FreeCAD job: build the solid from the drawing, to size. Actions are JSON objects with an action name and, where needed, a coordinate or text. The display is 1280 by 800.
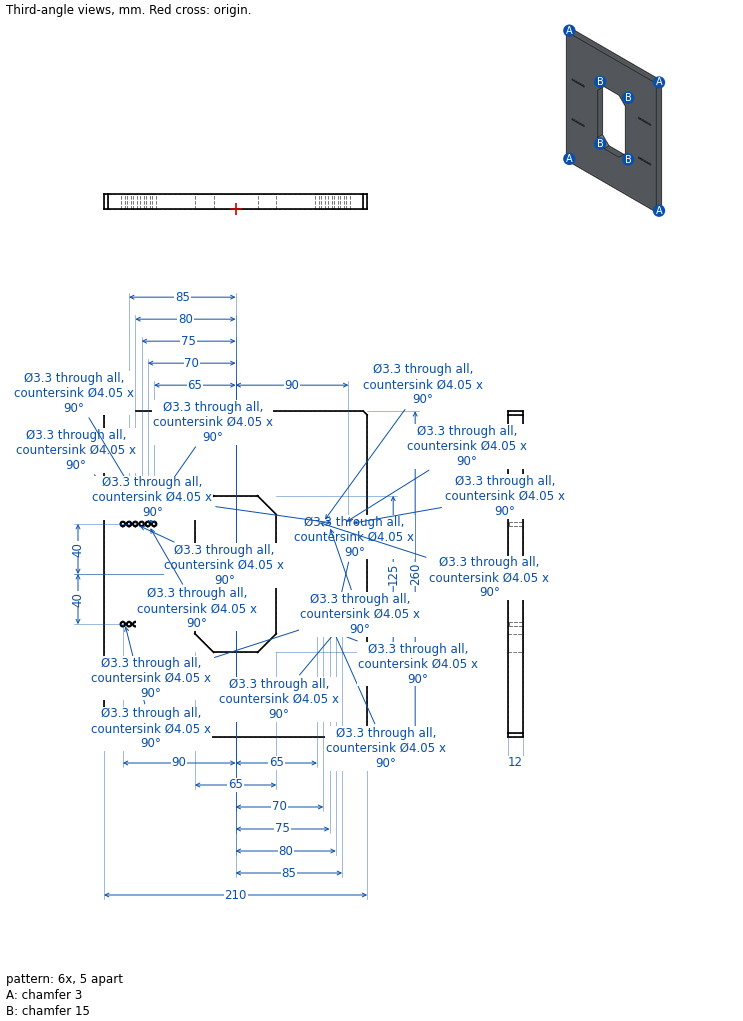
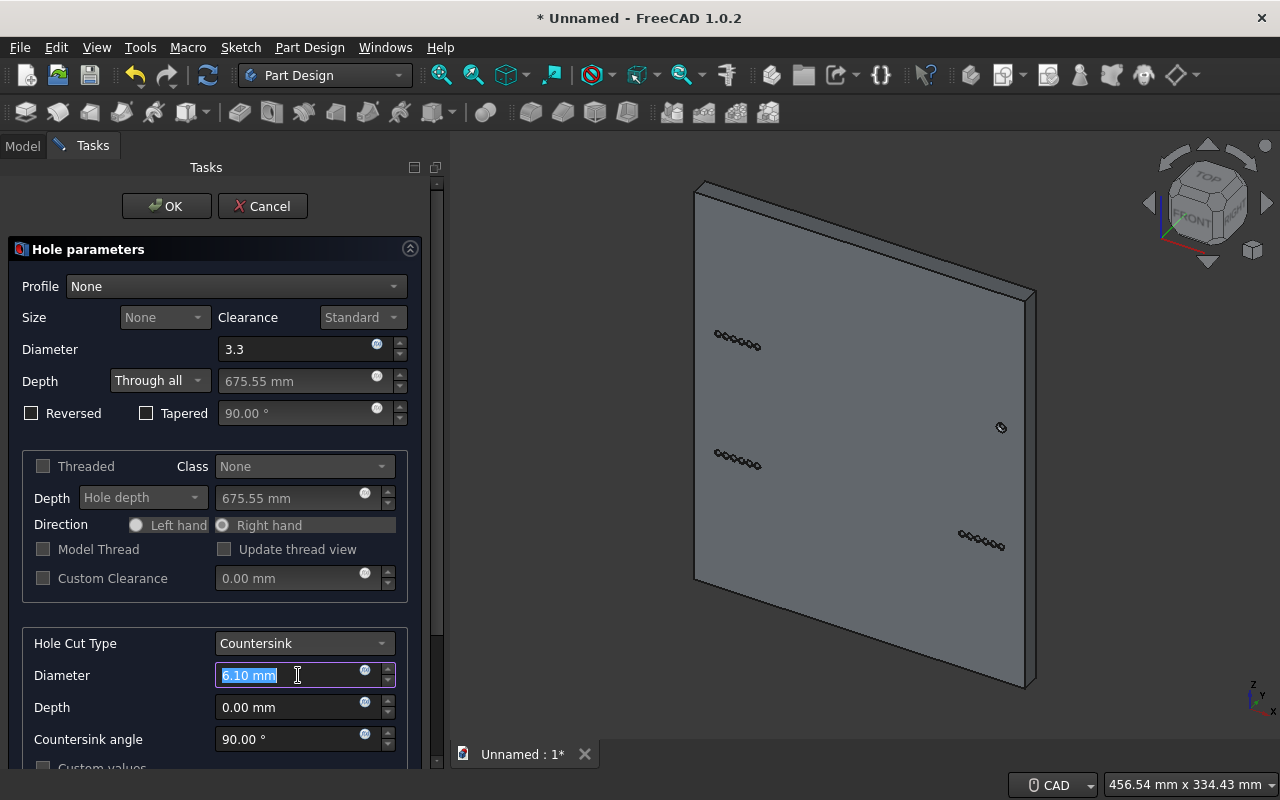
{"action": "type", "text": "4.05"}
{"action": "key", "text": "Tab"}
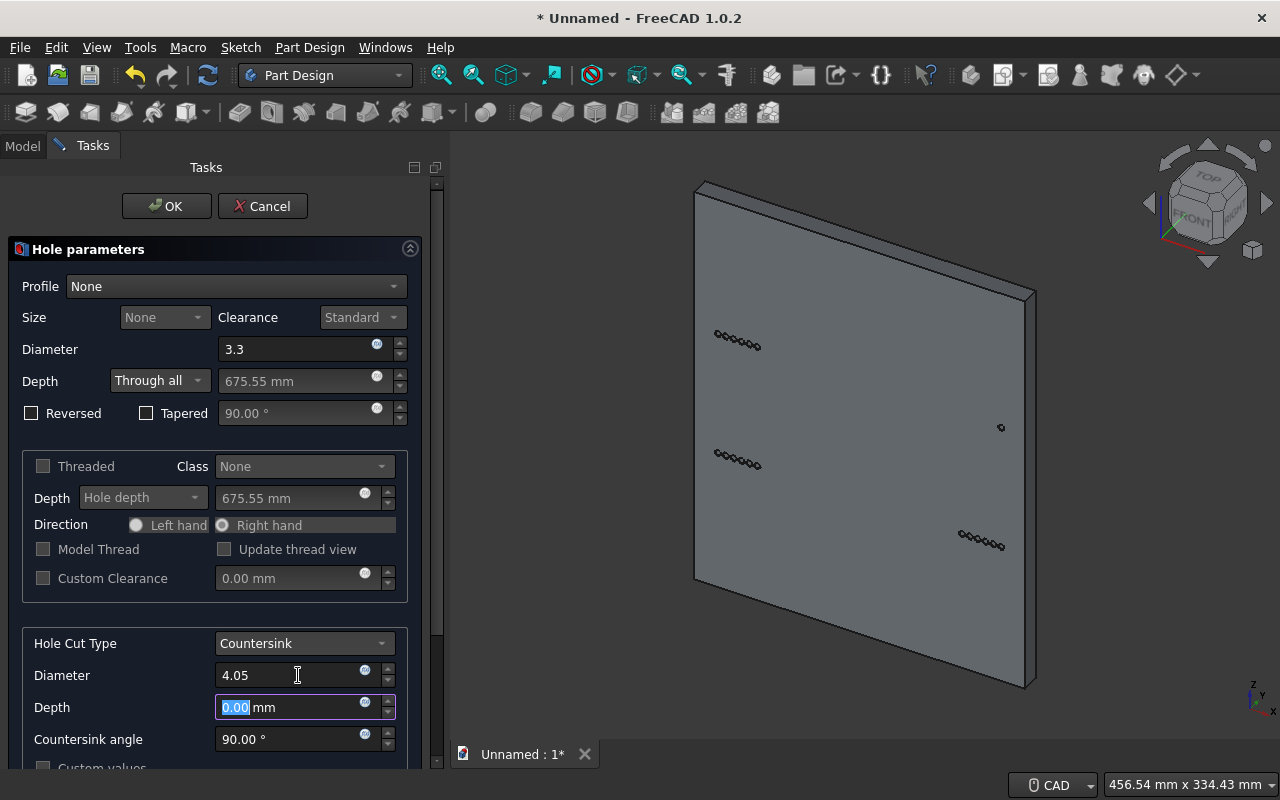
{"action": "left_click", "coordinate": [167, 206]}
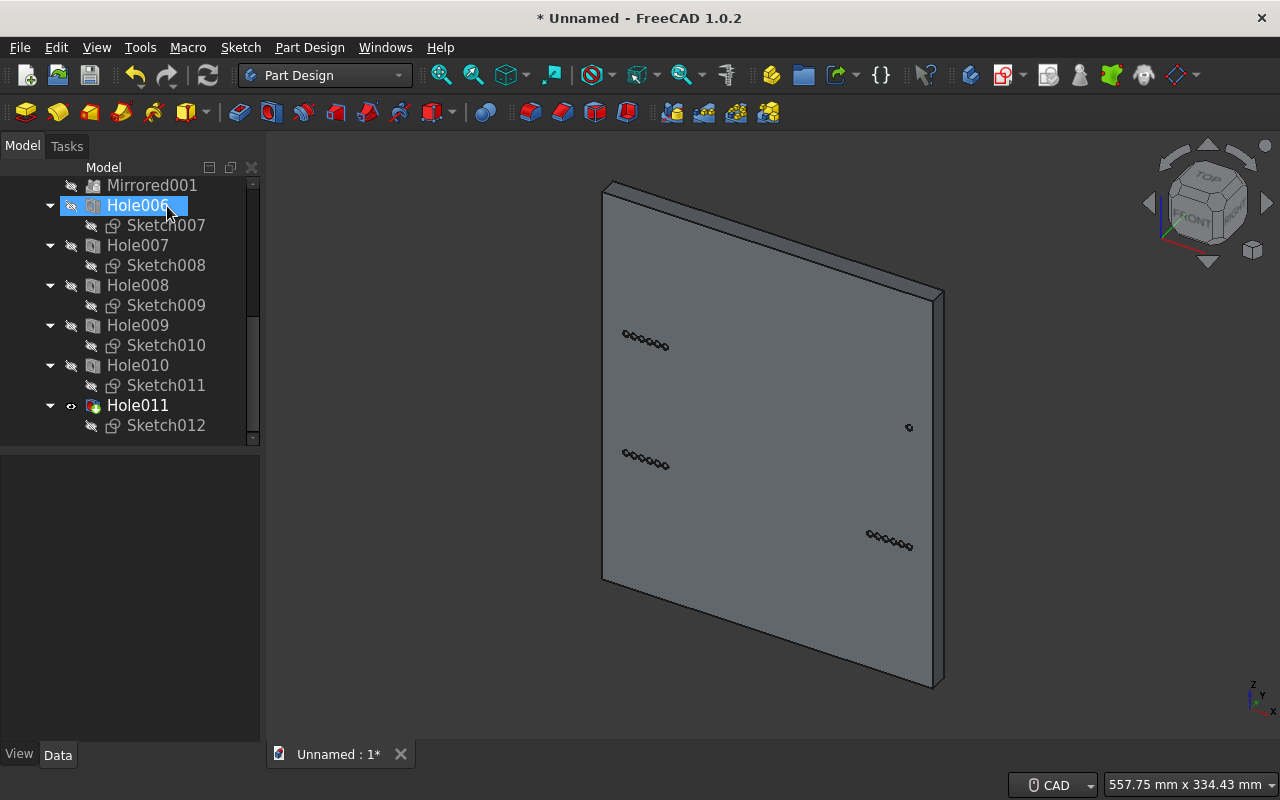
{"action": "left_click", "coordinate": [1004, 76]}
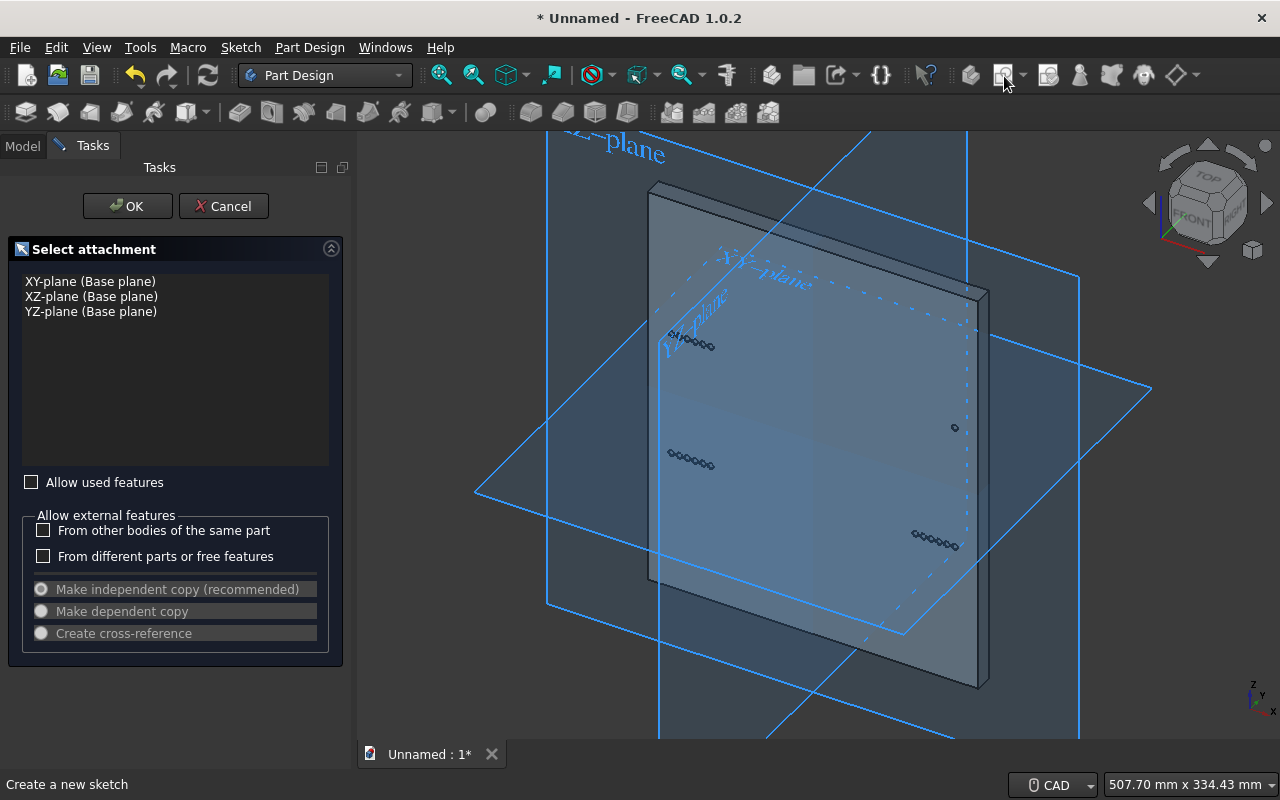
{"action": "left_click", "coordinate": [82, 296]}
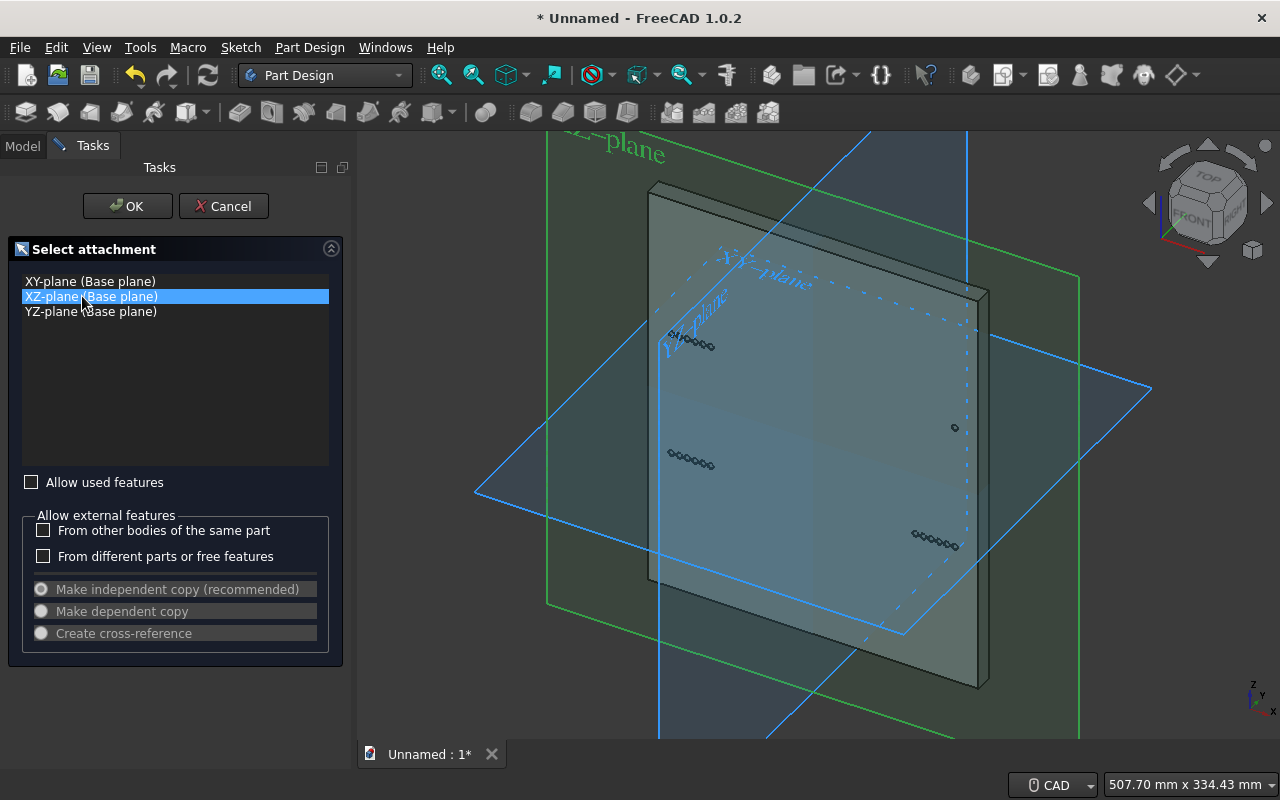
{"action": "left_click", "coordinate": [128, 206]}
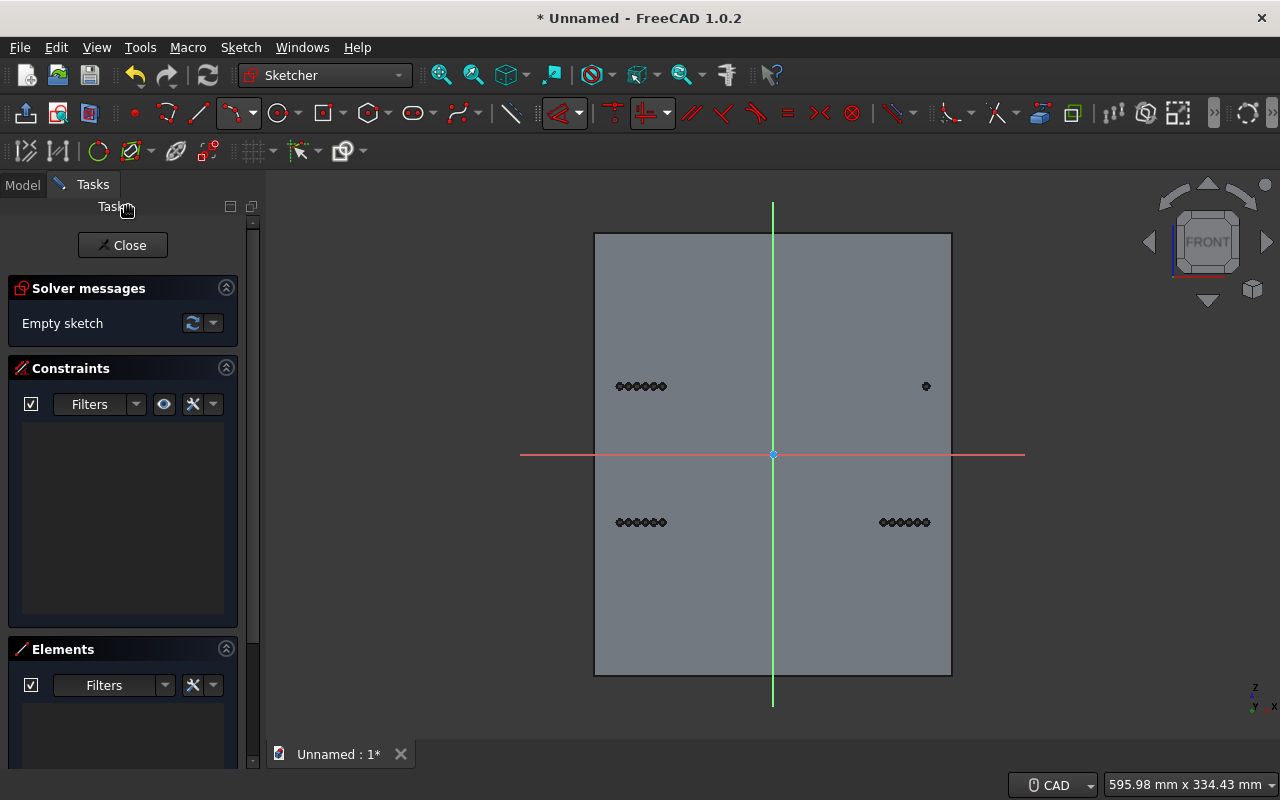
{"action": "scroll", "coordinate": [929, 383], "scroll_direction": "up", "scroll_amount": 15}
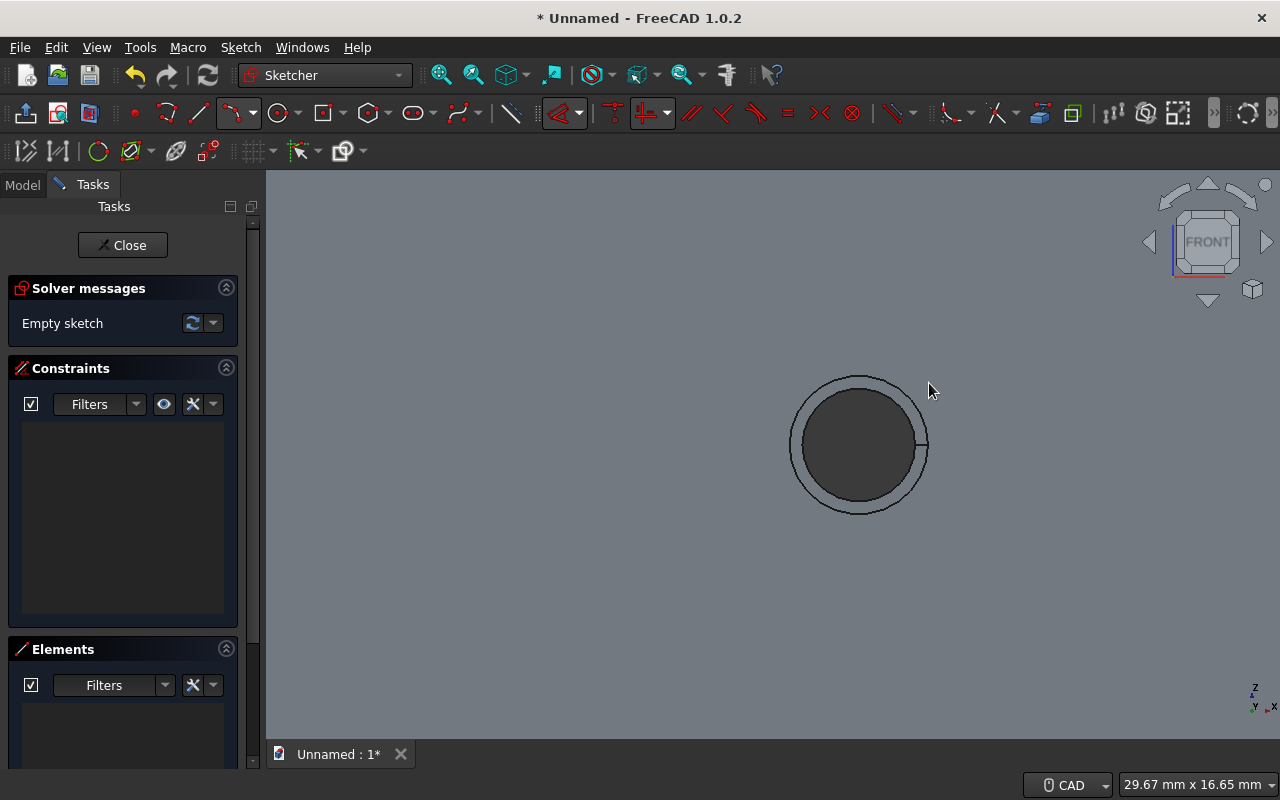
{"action": "scroll", "coordinate": [681, 441], "scroll_direction": "up", "scroll_amount": 6}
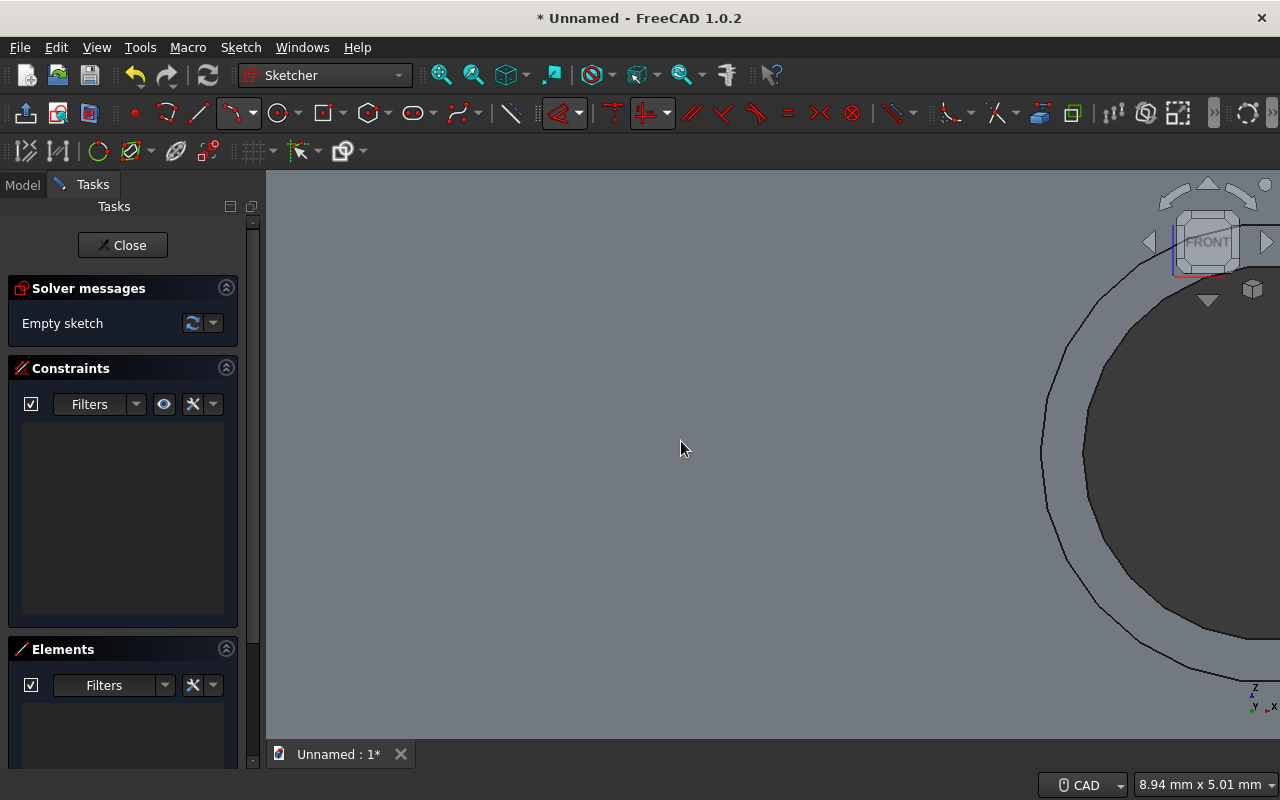
{"action": "left_click", "coordinate": [278, 114]}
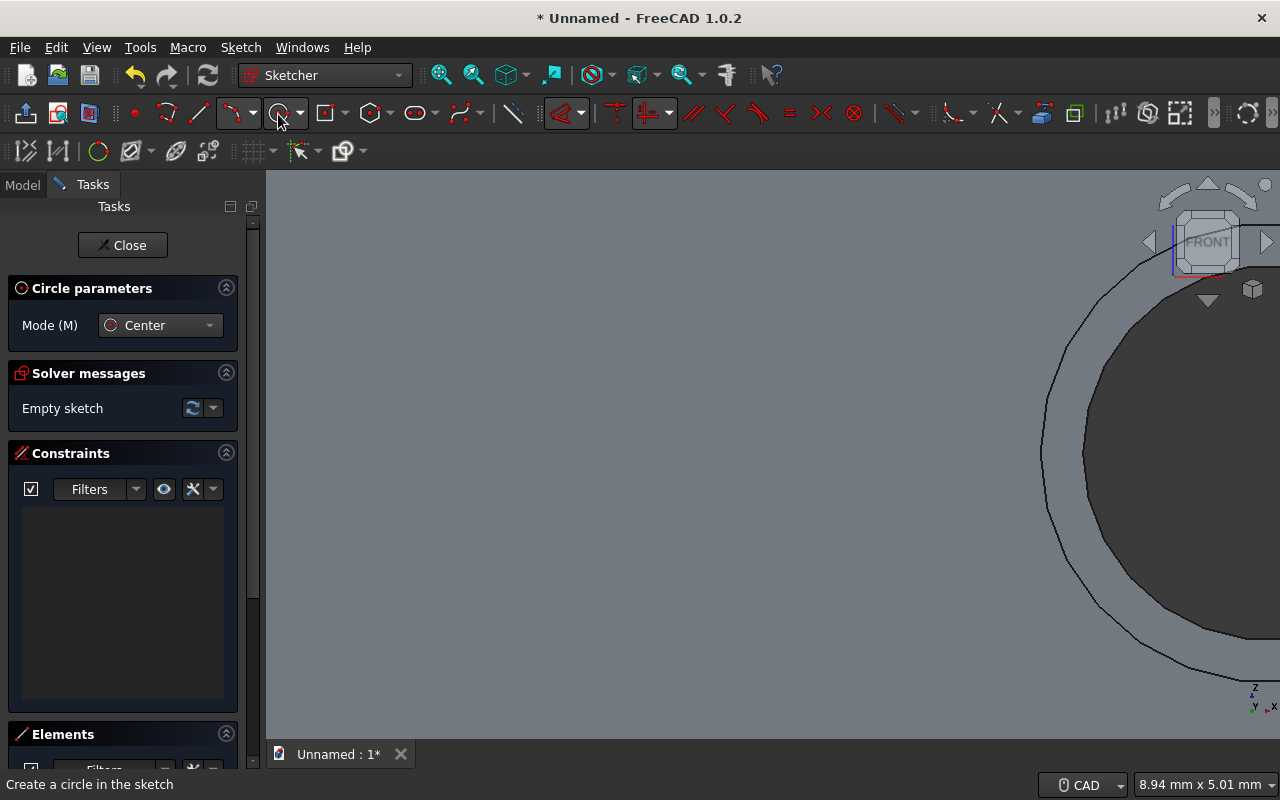
{"action": "left_click", "coordinate": [703, 453]}
{"action": "mouse_move", "coordinate": [835, 321]}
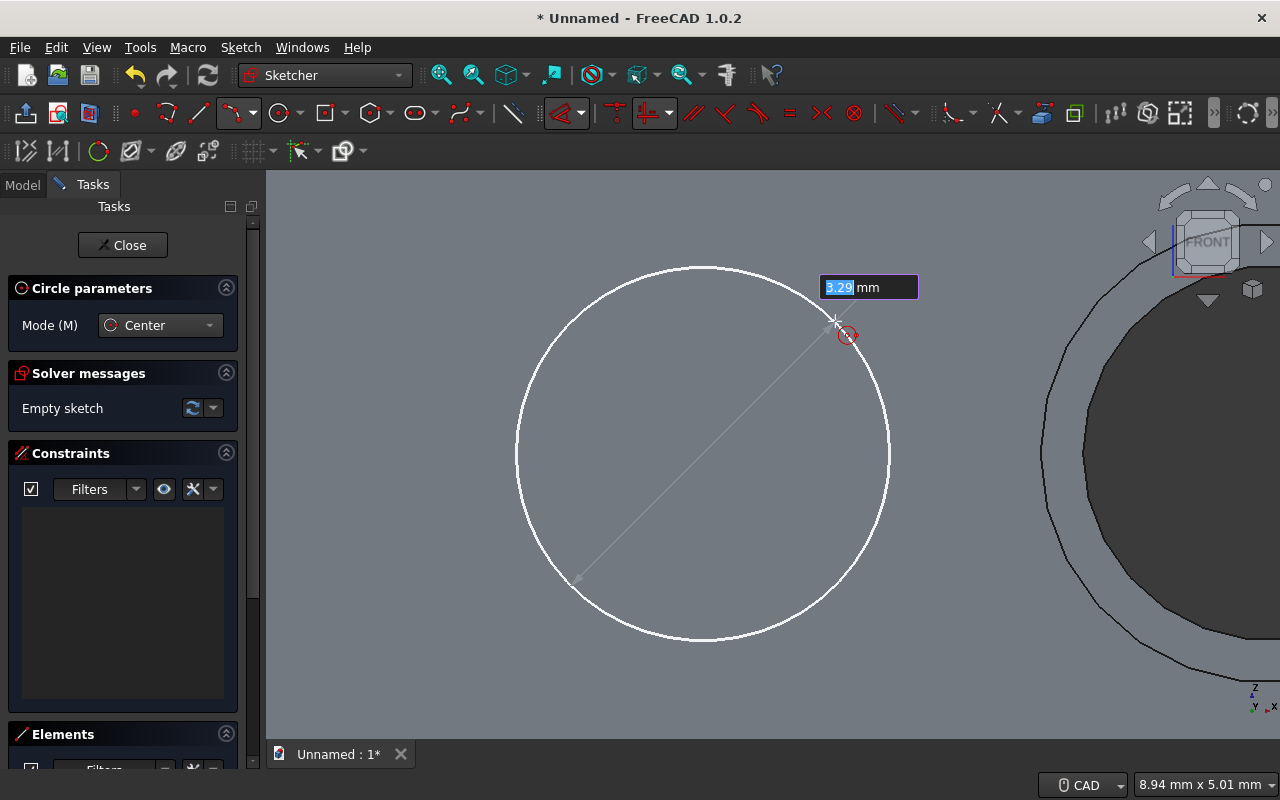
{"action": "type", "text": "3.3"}
{"action": "key", "text": "Return"}
{"action": "key", "text": "Escape"}